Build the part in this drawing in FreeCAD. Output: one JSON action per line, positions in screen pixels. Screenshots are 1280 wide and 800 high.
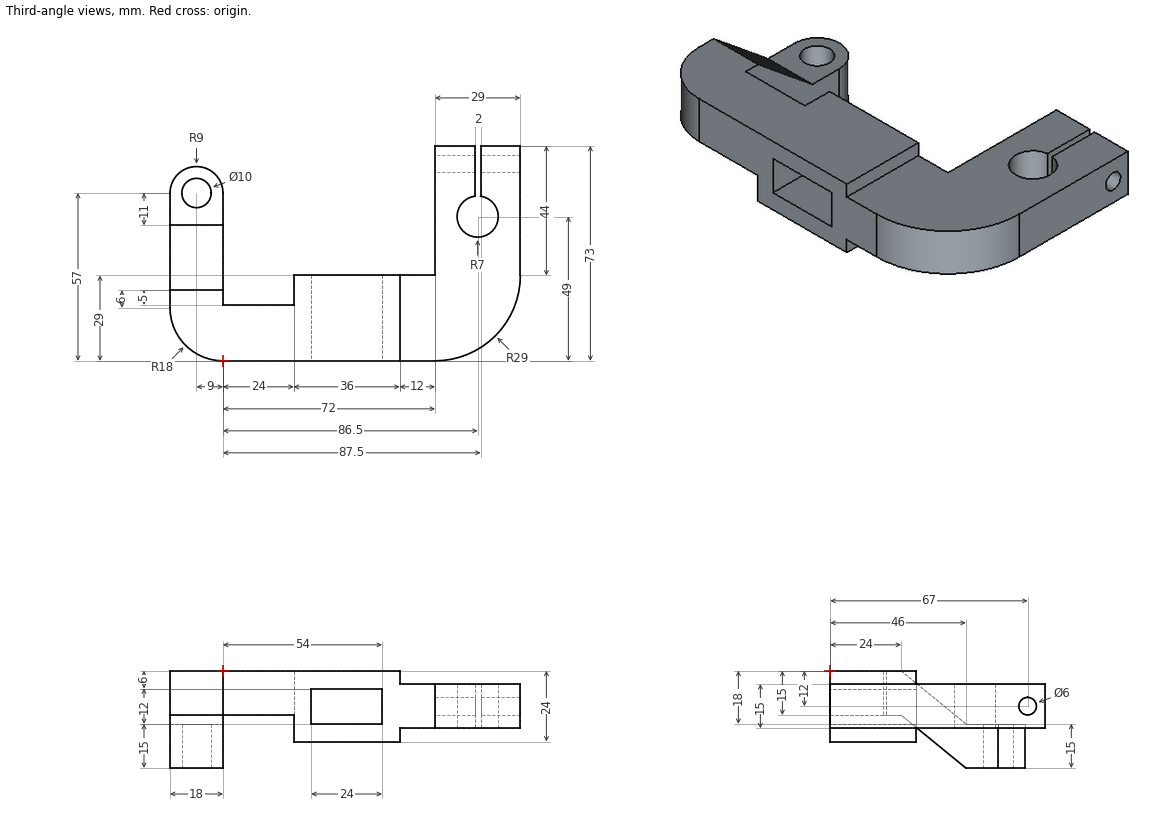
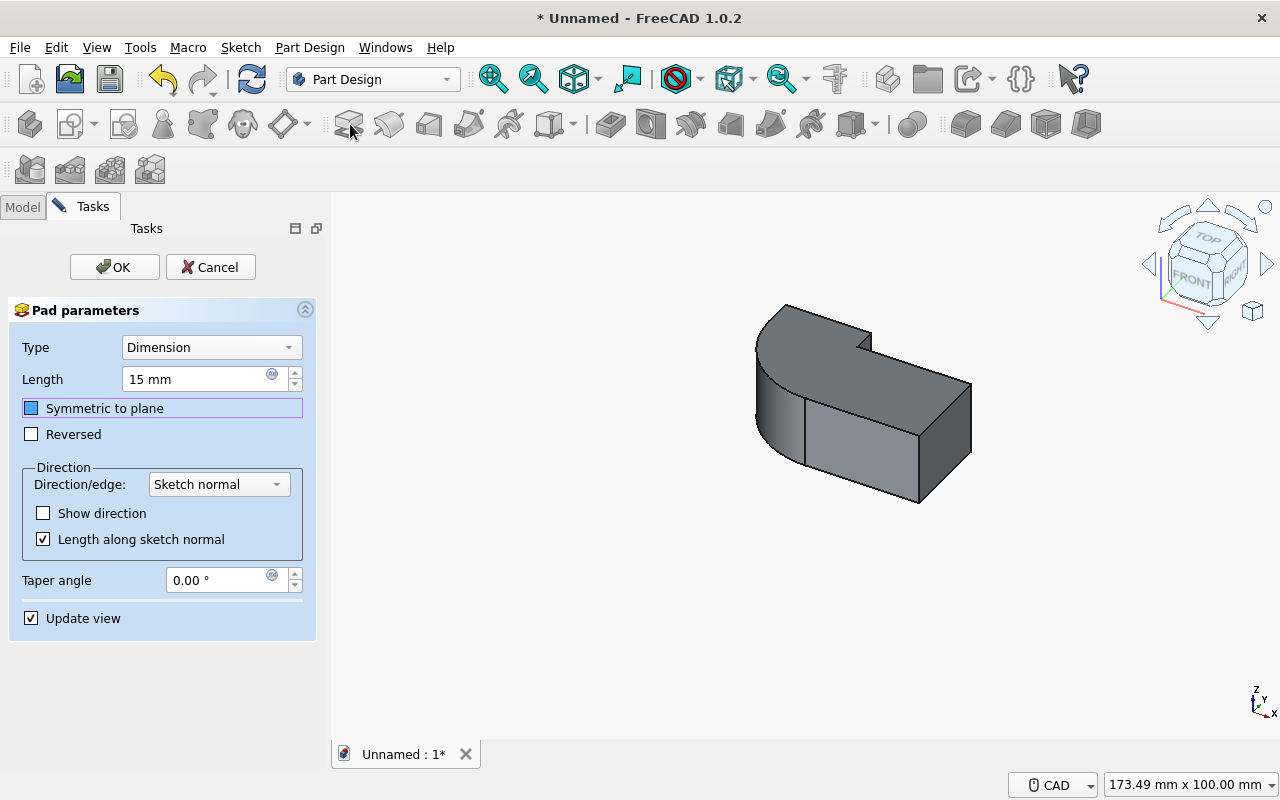
{"action": "left_click", "coordinate": [30, 434]}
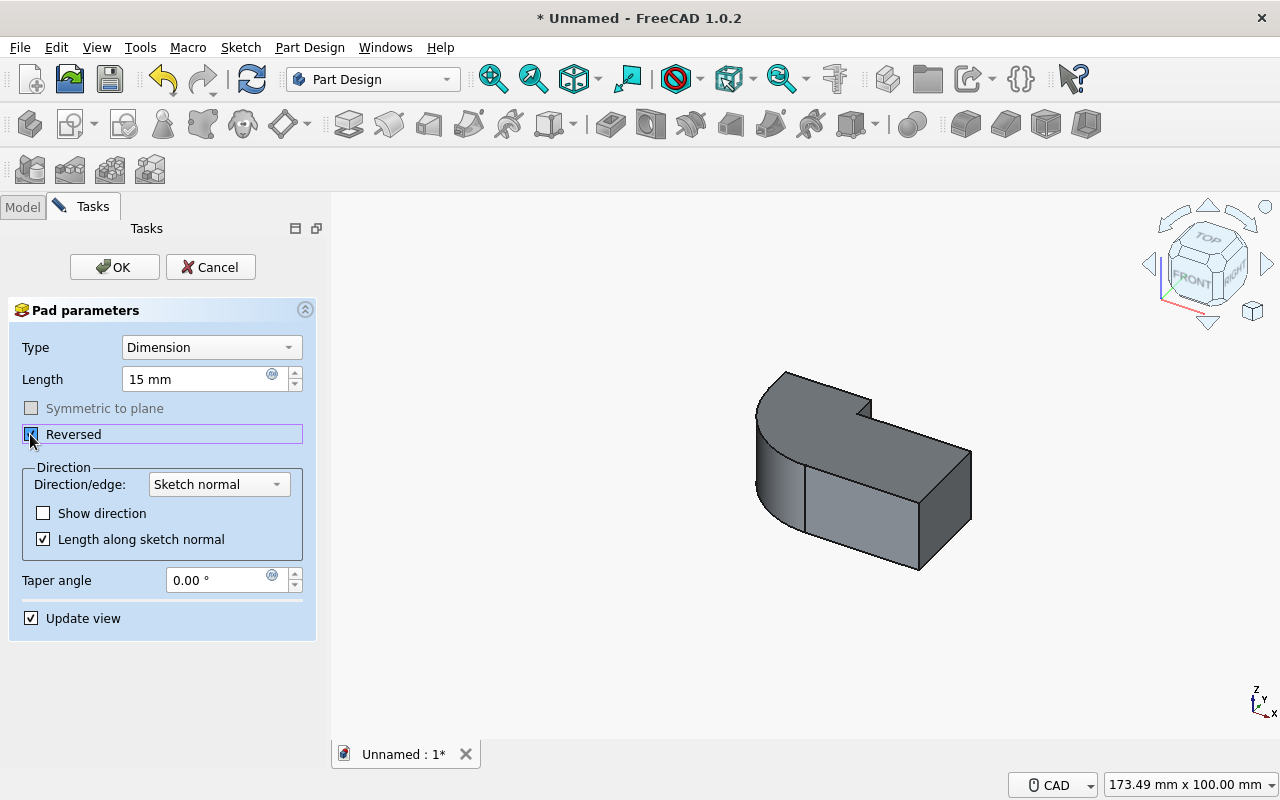
{"action": "left_click", "coordinate": [115, 267]}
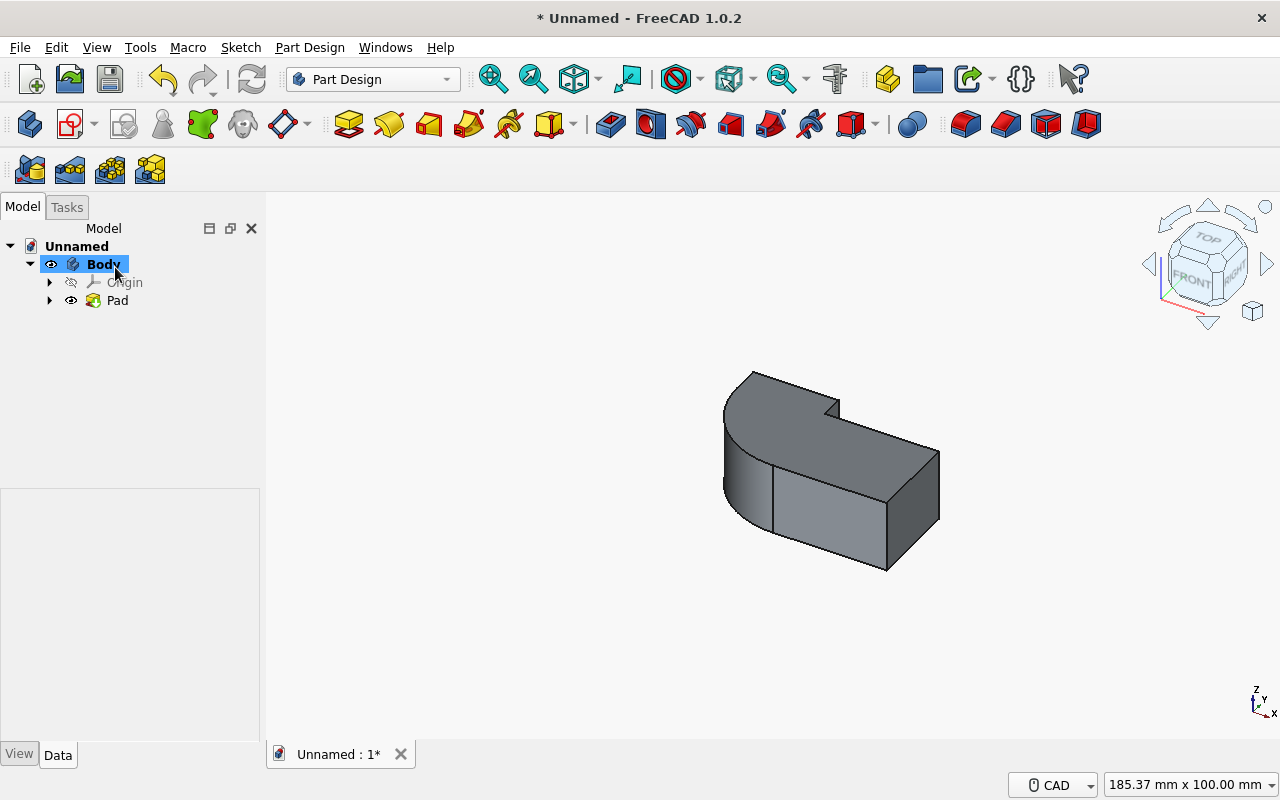
{"action": "left_click", "coordinate": [494, 80]}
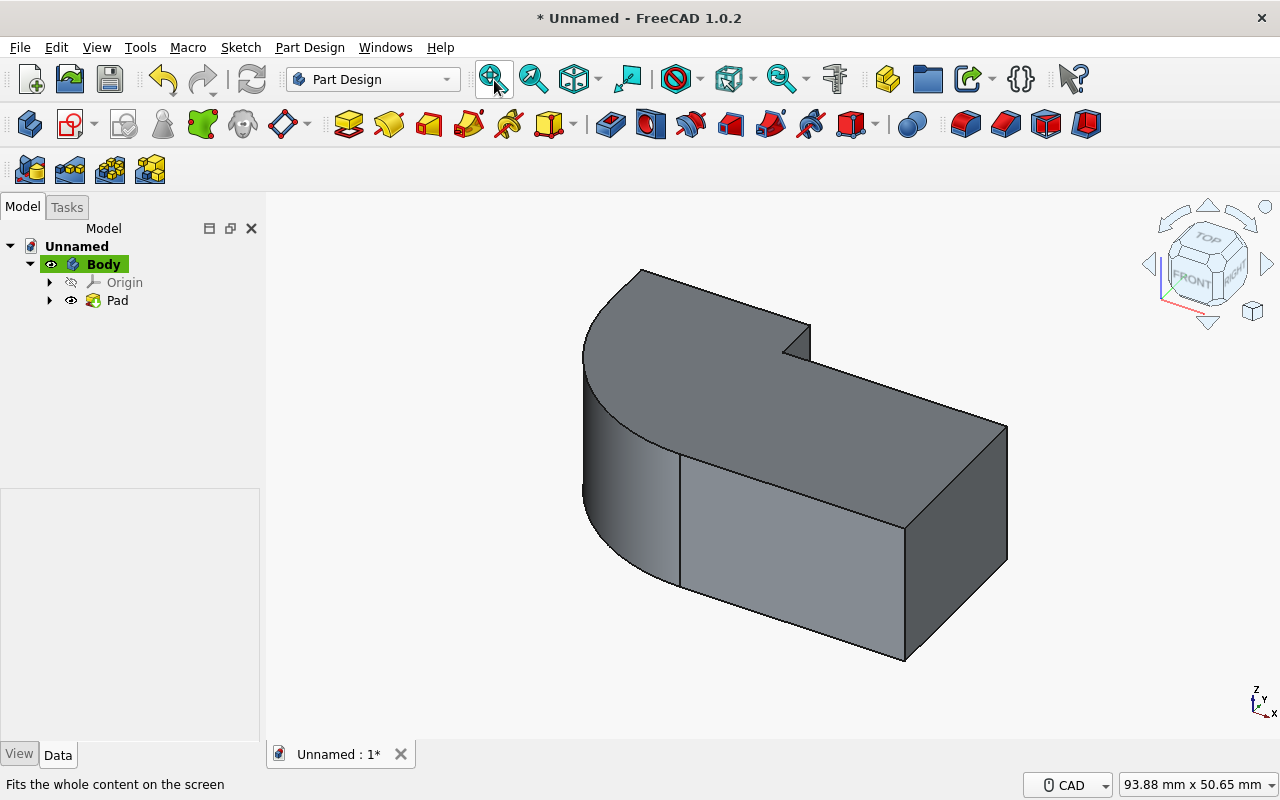
{"action": "left_click", "coordinate": [867, 454]}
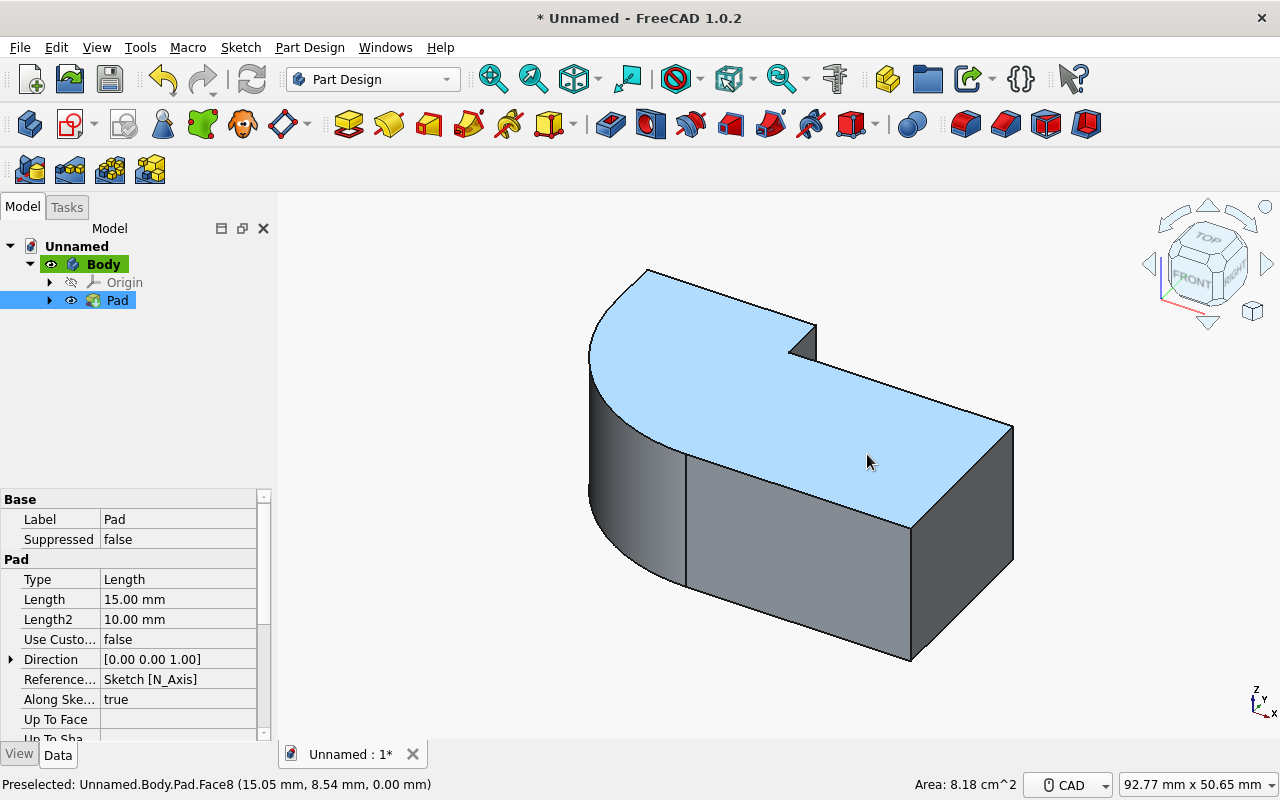
{"action": "left_click", "coordinate": [70, 124]}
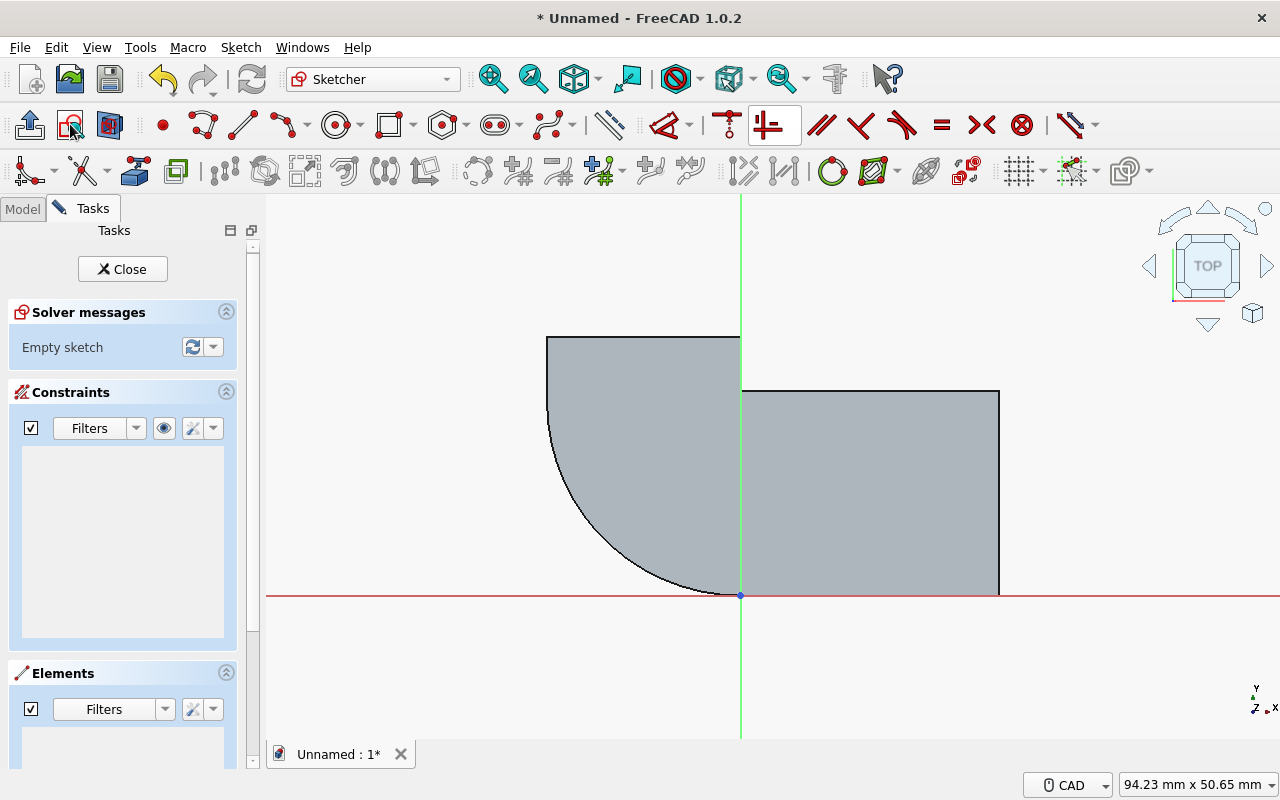
{"action": "scroll", "coordinate": [294, 521], "scroll_direction": "down", "scroll_amount": 2}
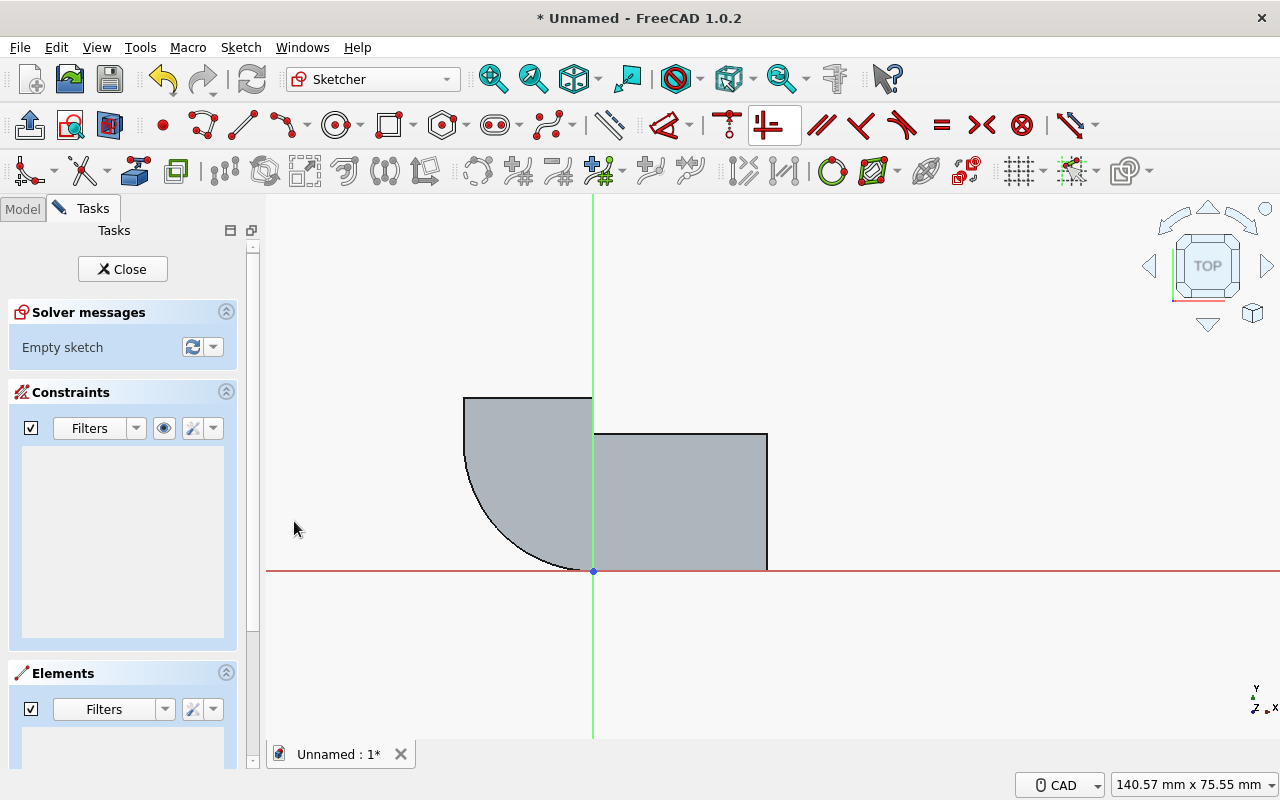
{"action": "left_click", "coordinate": [390, 126]}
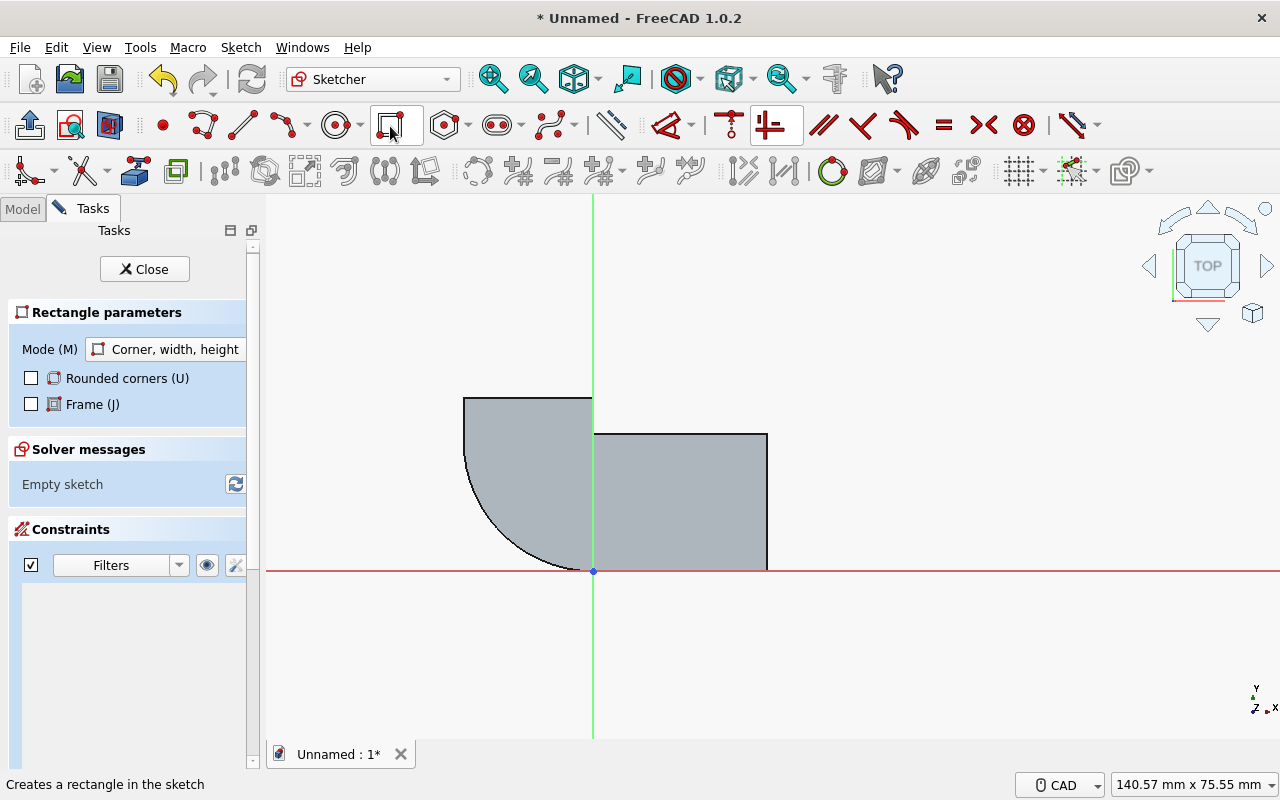
{"action": "left_click", "coordinate": [767, 362]}
{"action": "left_click", "coordinate": [1026, 571]}
{"action": "key", "text": "Escape"}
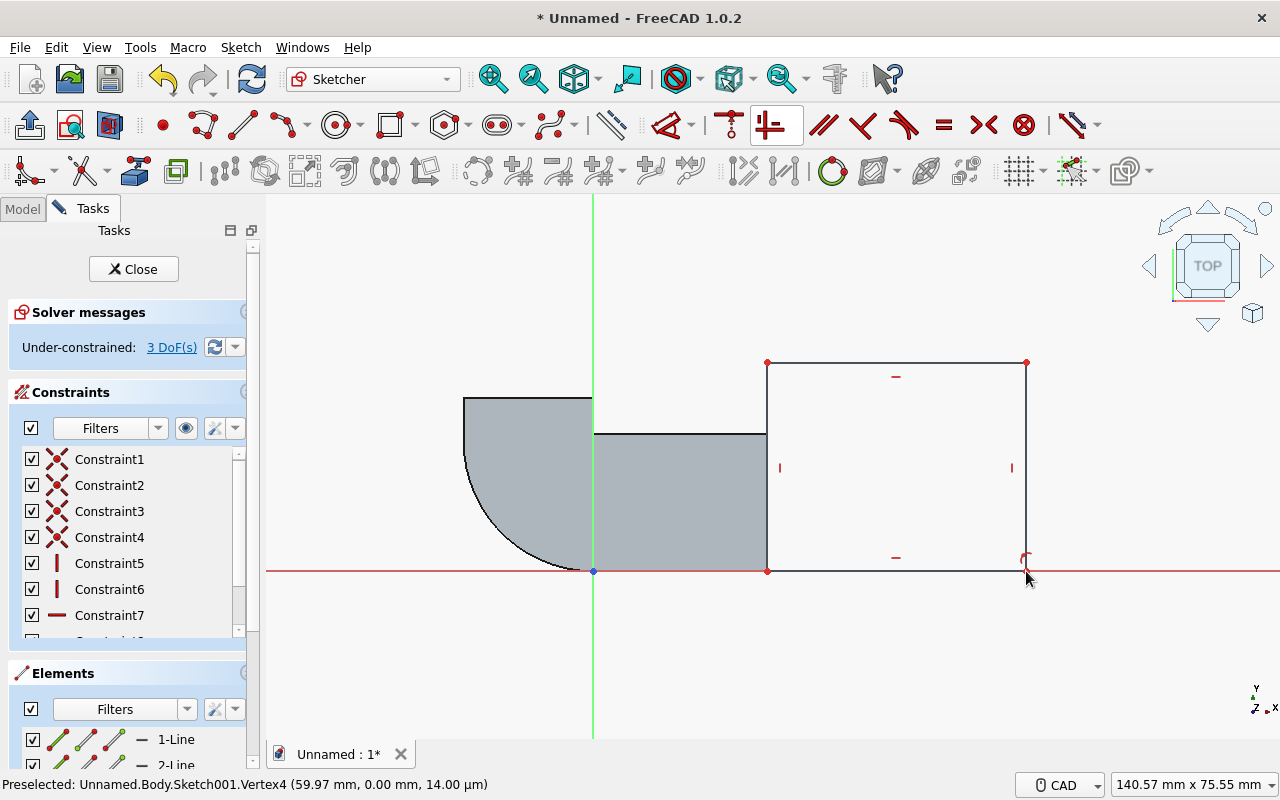
{"action": "left_click", "coordinate": [666, 126]}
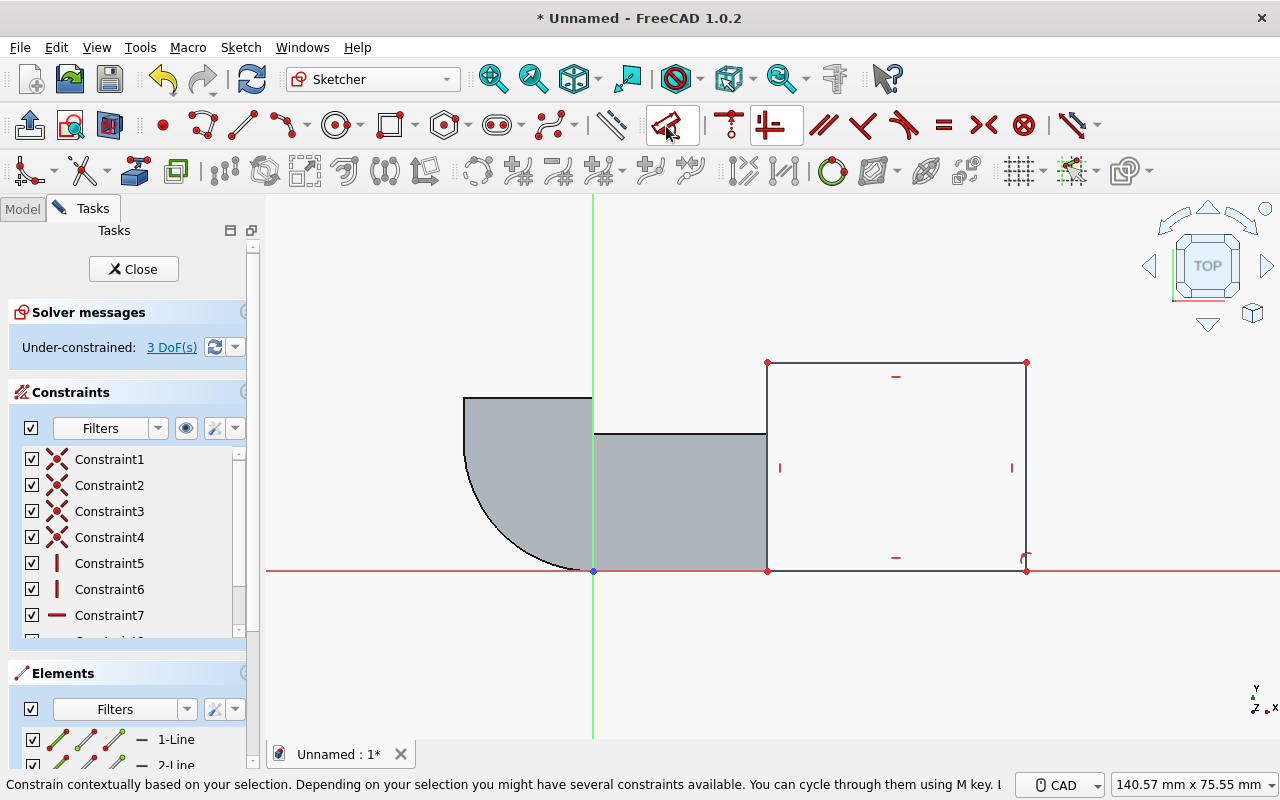
{"action": "left_click", "coordinate": [767, 425]}
{"action": "left_click", "coordinate": [733, 467]}